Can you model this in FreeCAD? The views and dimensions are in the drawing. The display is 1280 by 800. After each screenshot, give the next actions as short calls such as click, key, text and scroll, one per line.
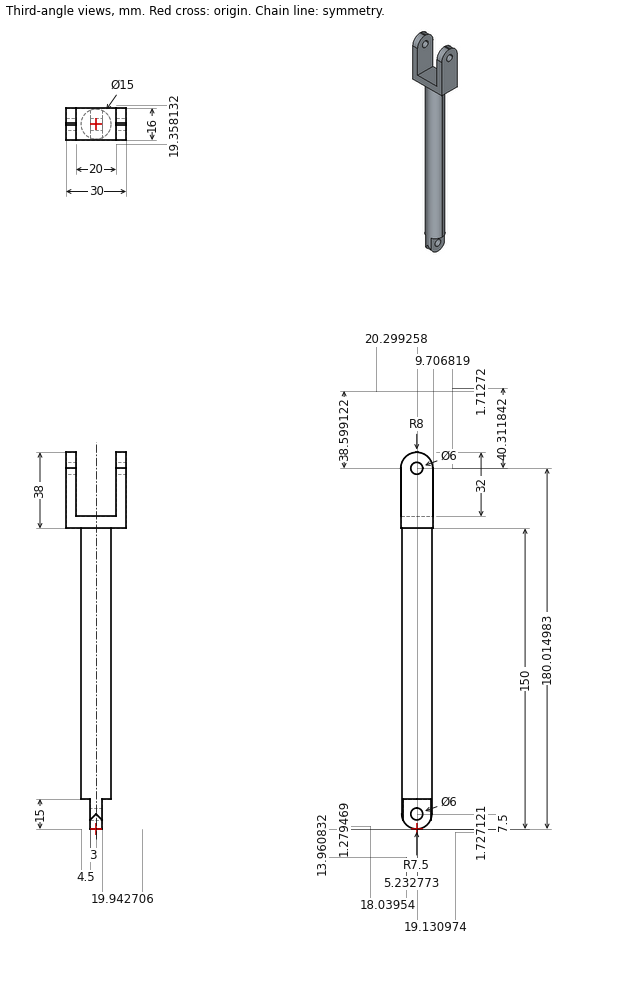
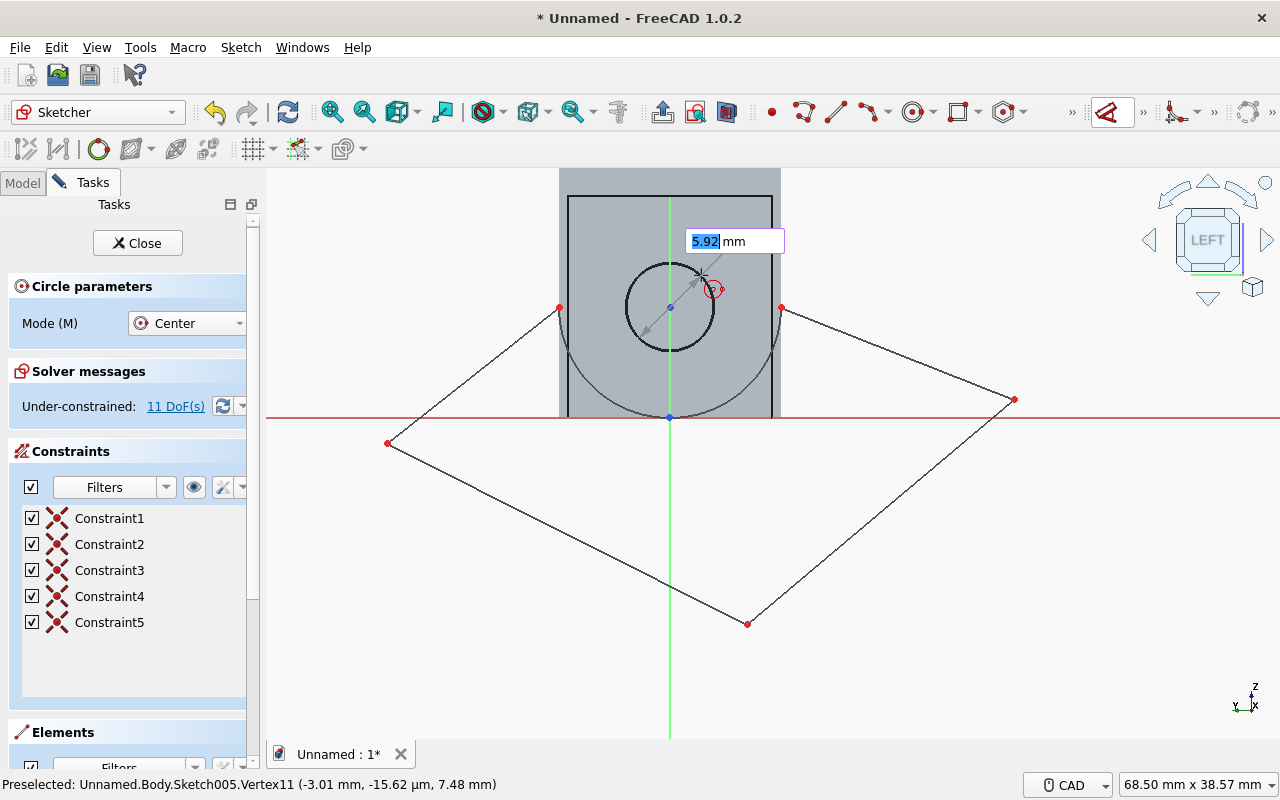
text(6)
key(Return)
key(Escape)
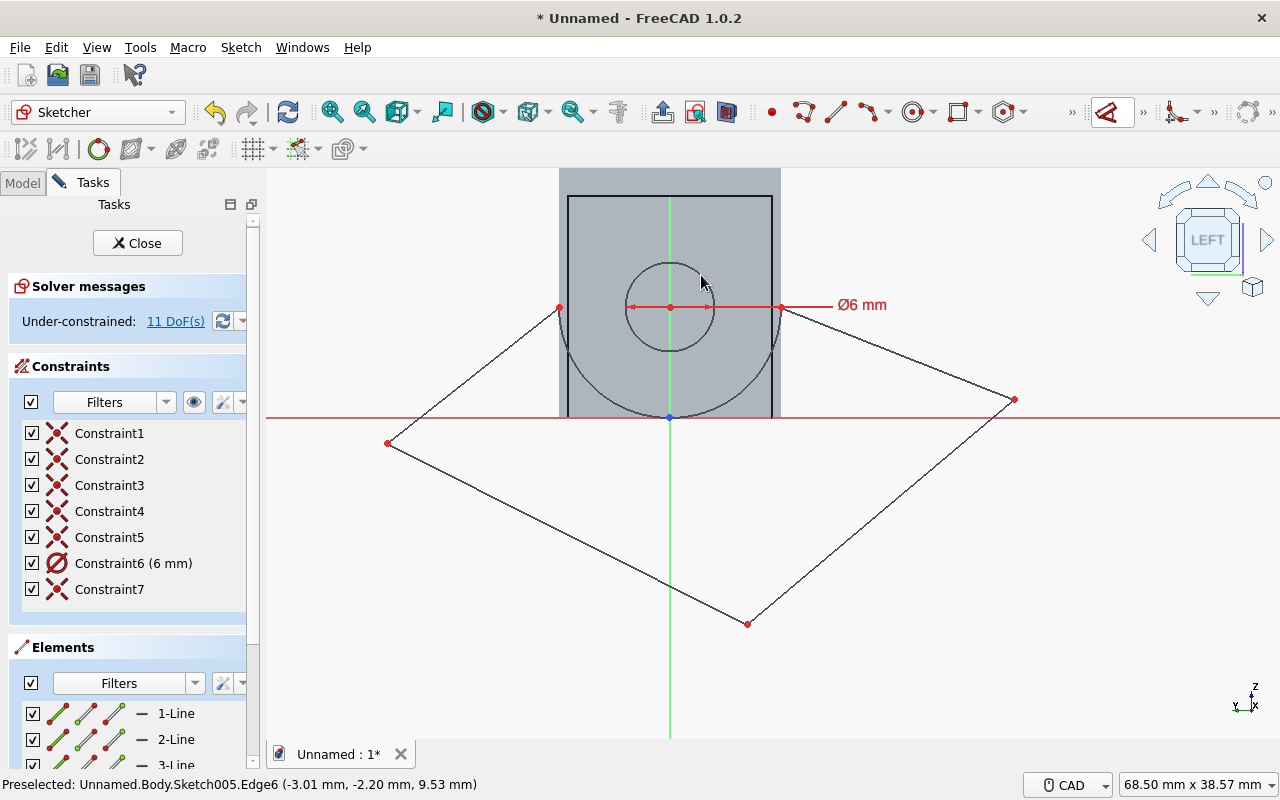
click(670, 307)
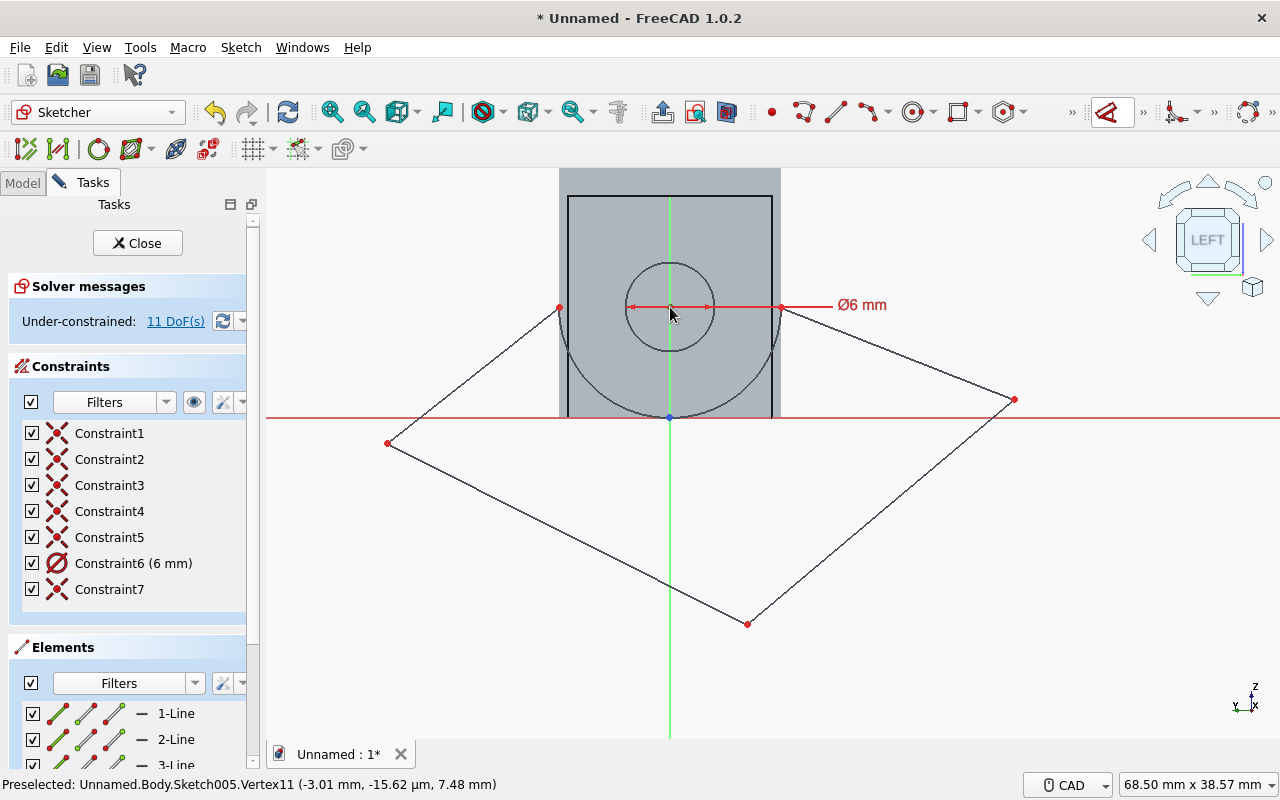
click(670, 674)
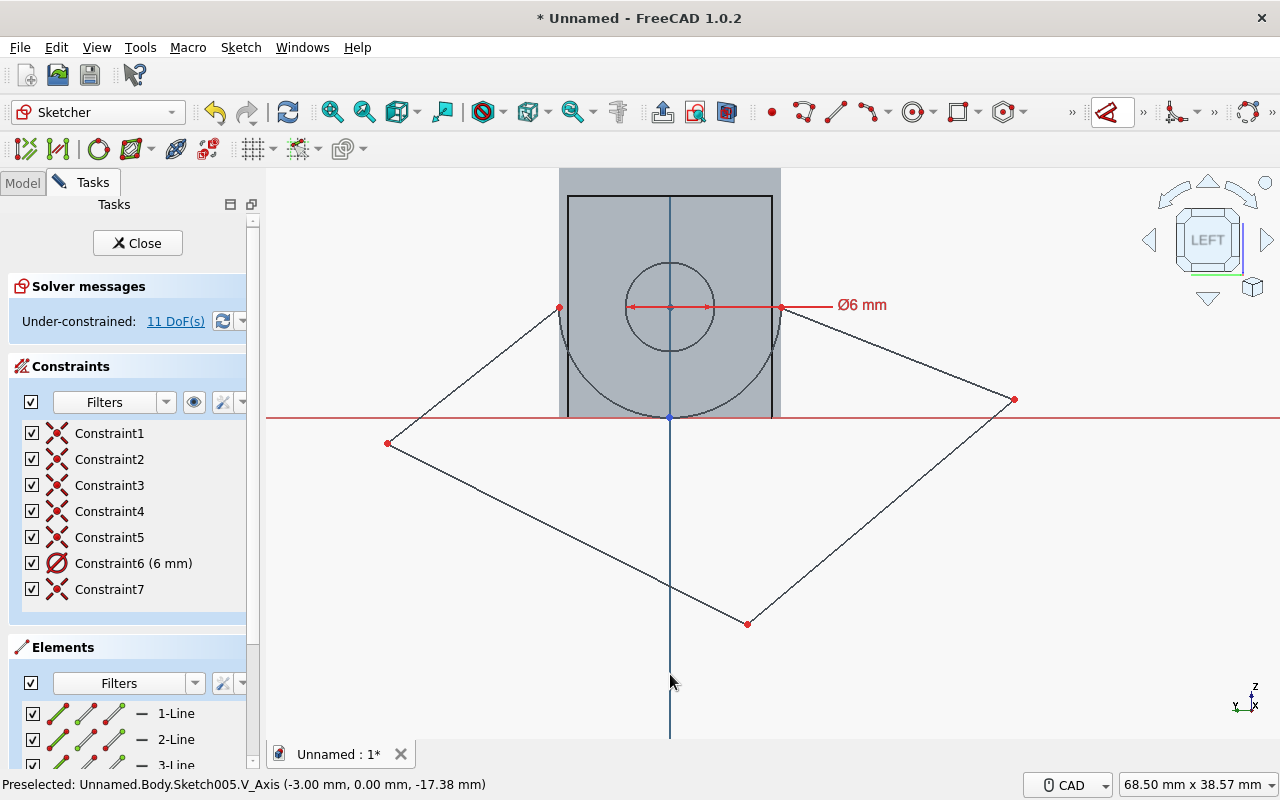
key(c)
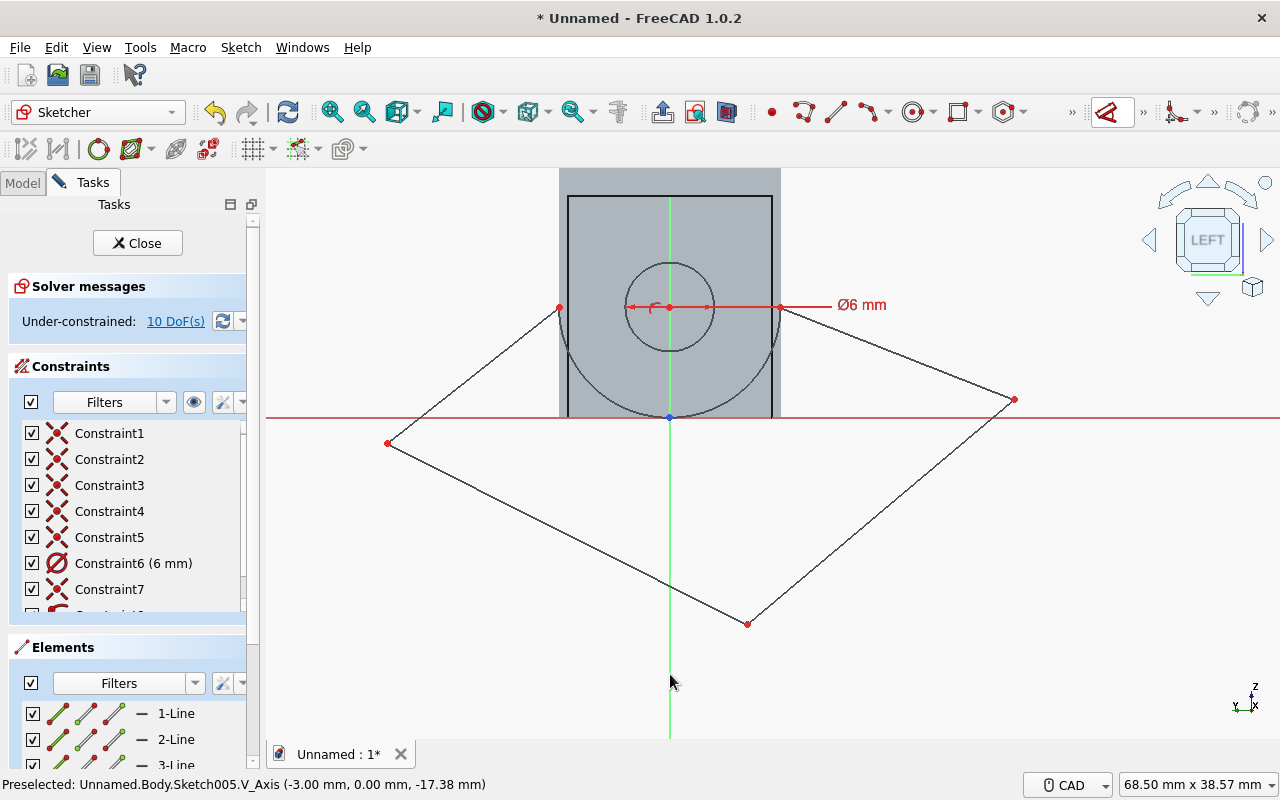
key(d)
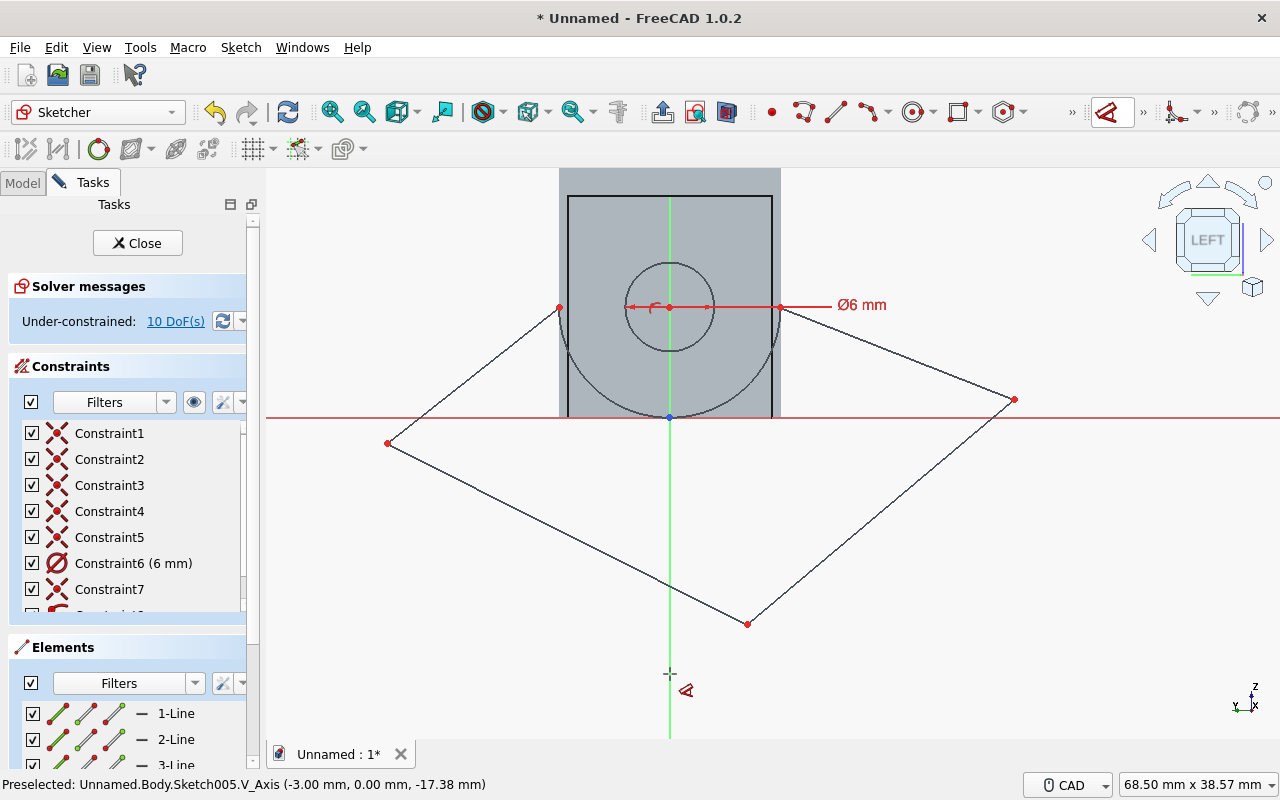
click(605, 397)
click(541, 369)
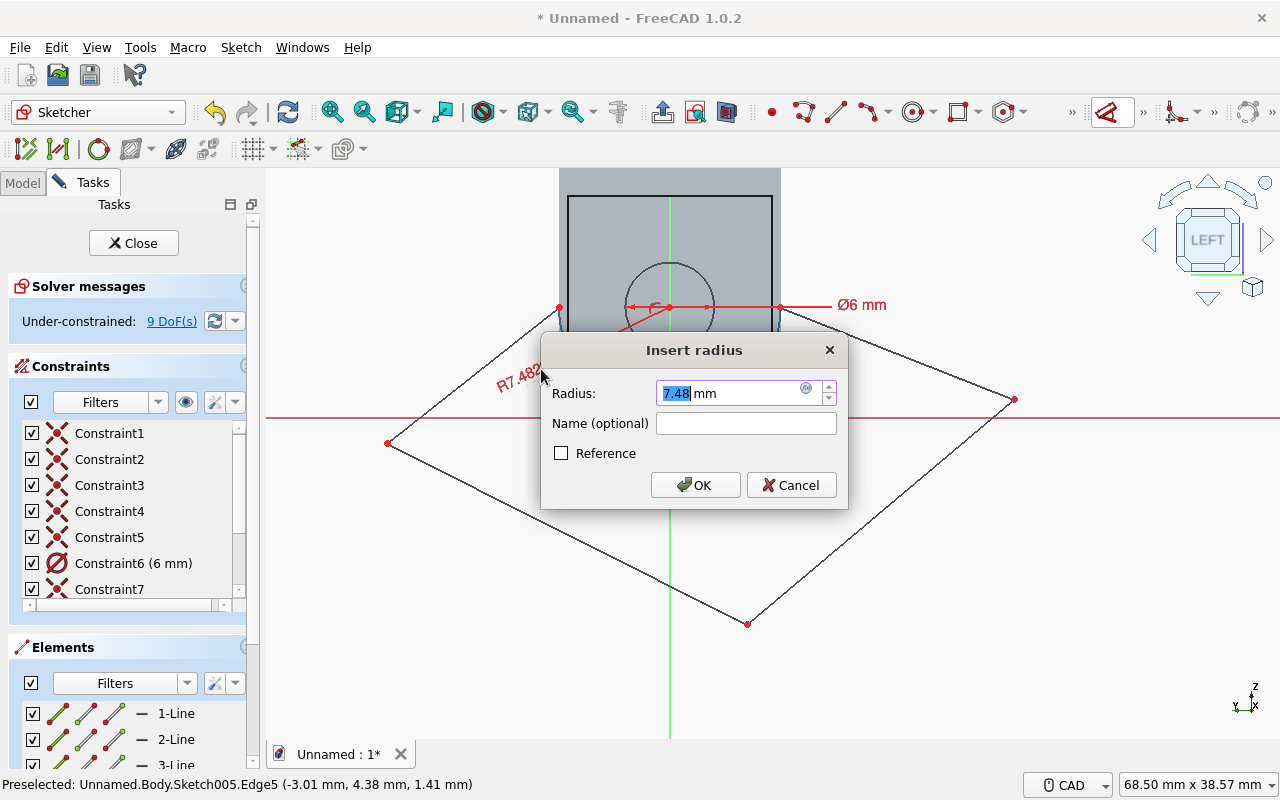
text(7.5)
key(Return)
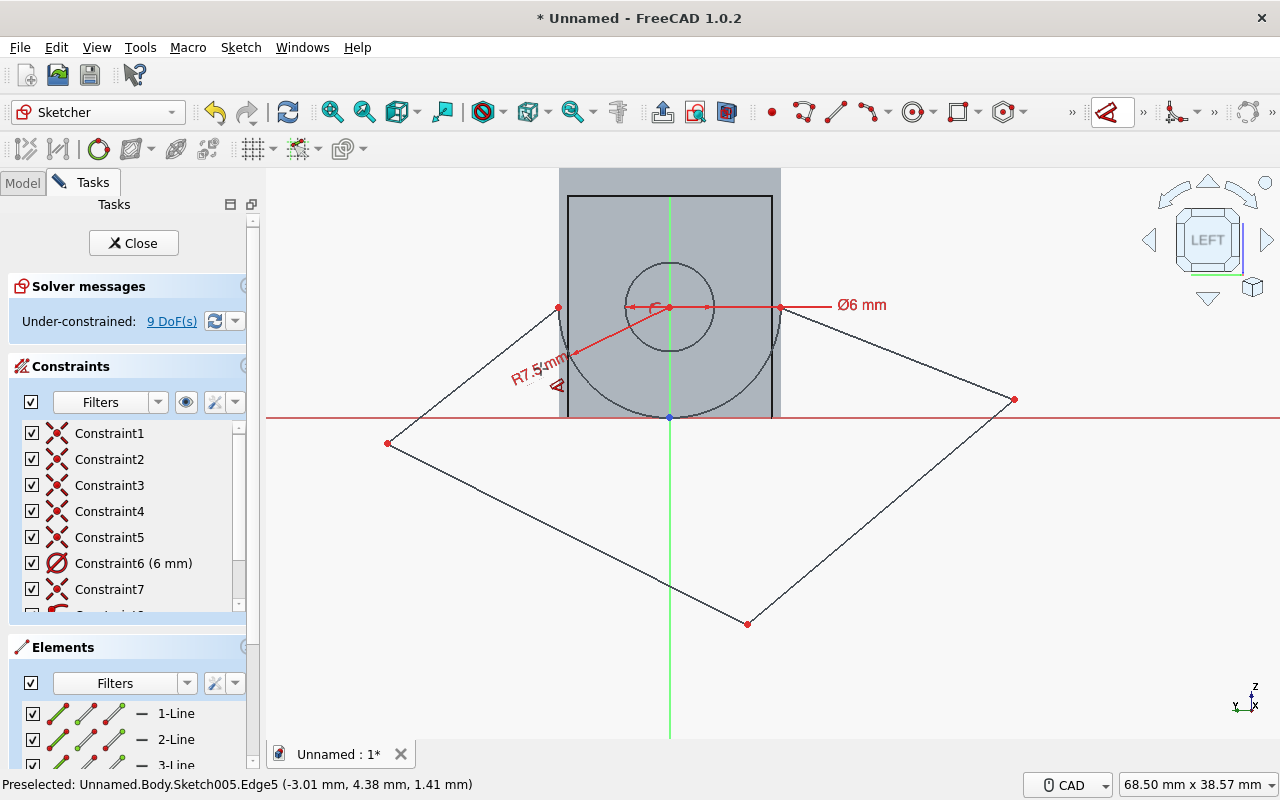
click(670, 307)
click(636, 362)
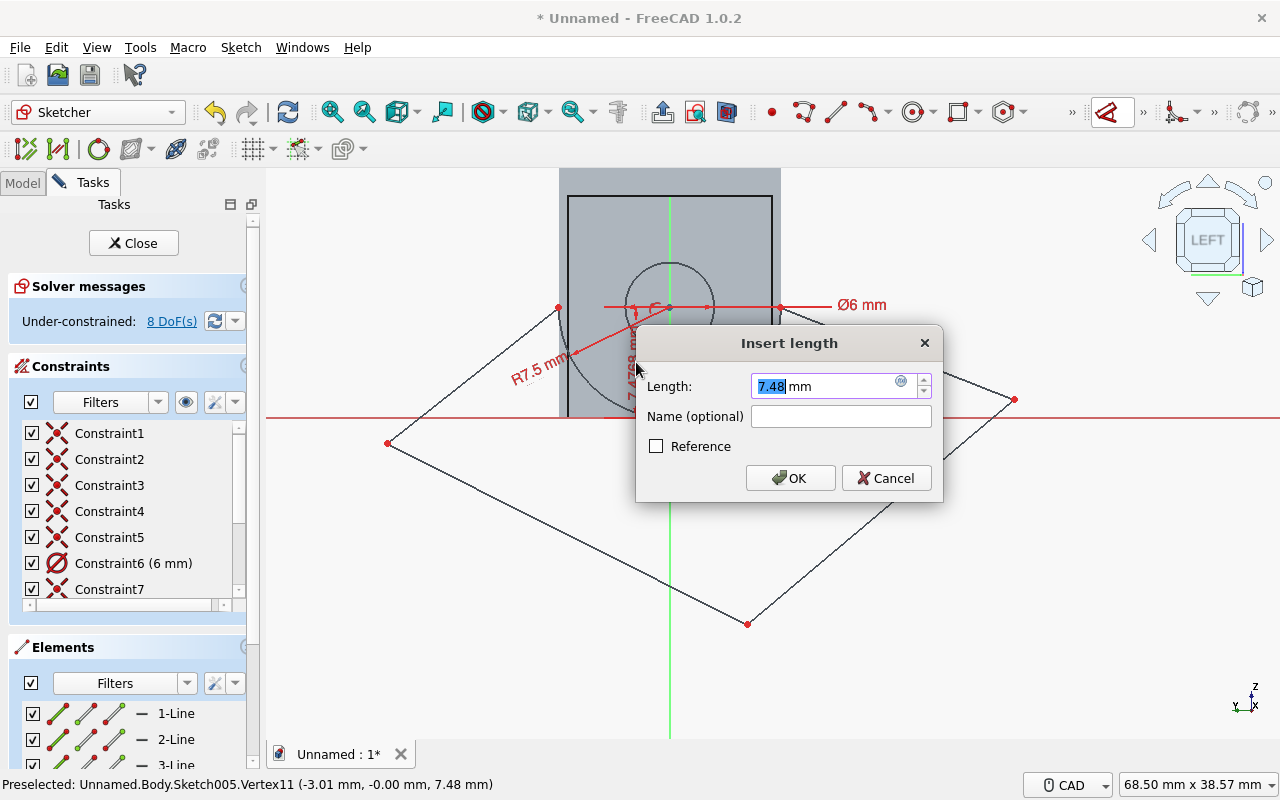
text(7.5)
key(Return)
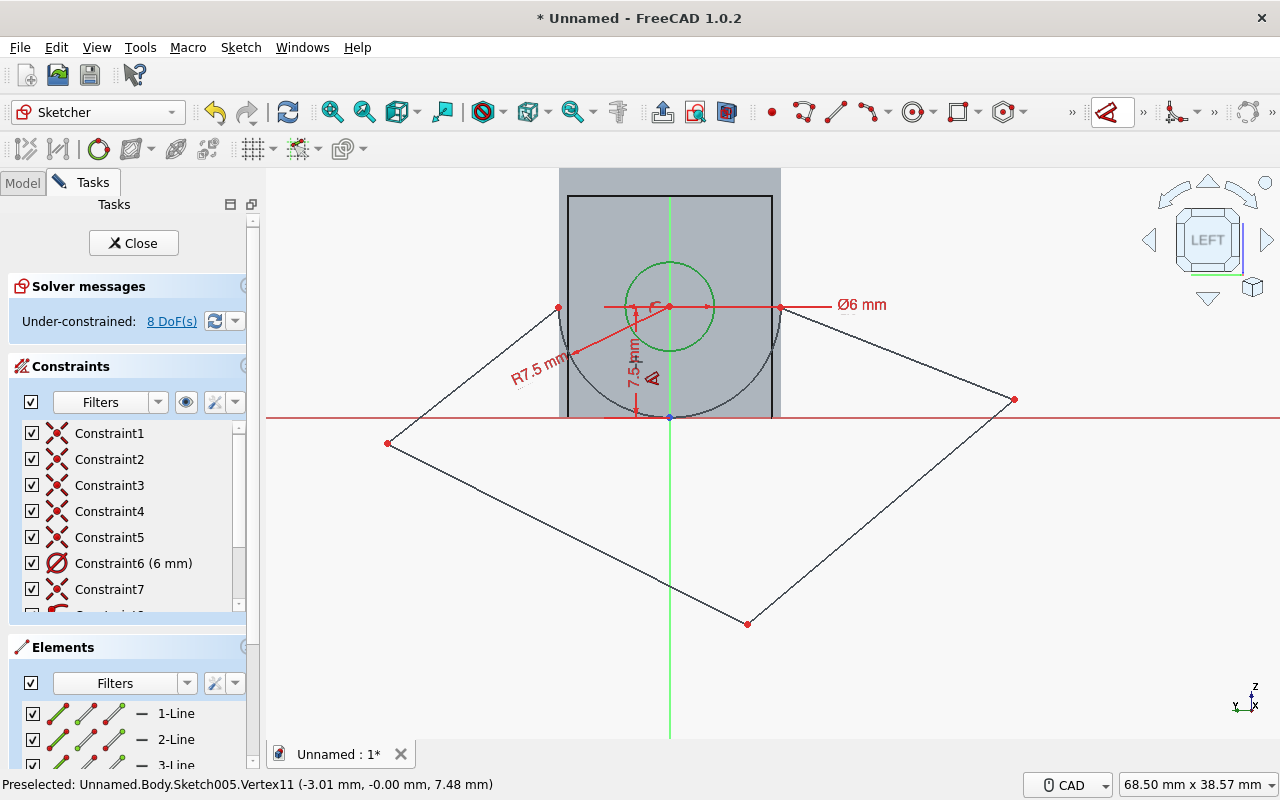
click(559, 308)
click(525, 401)